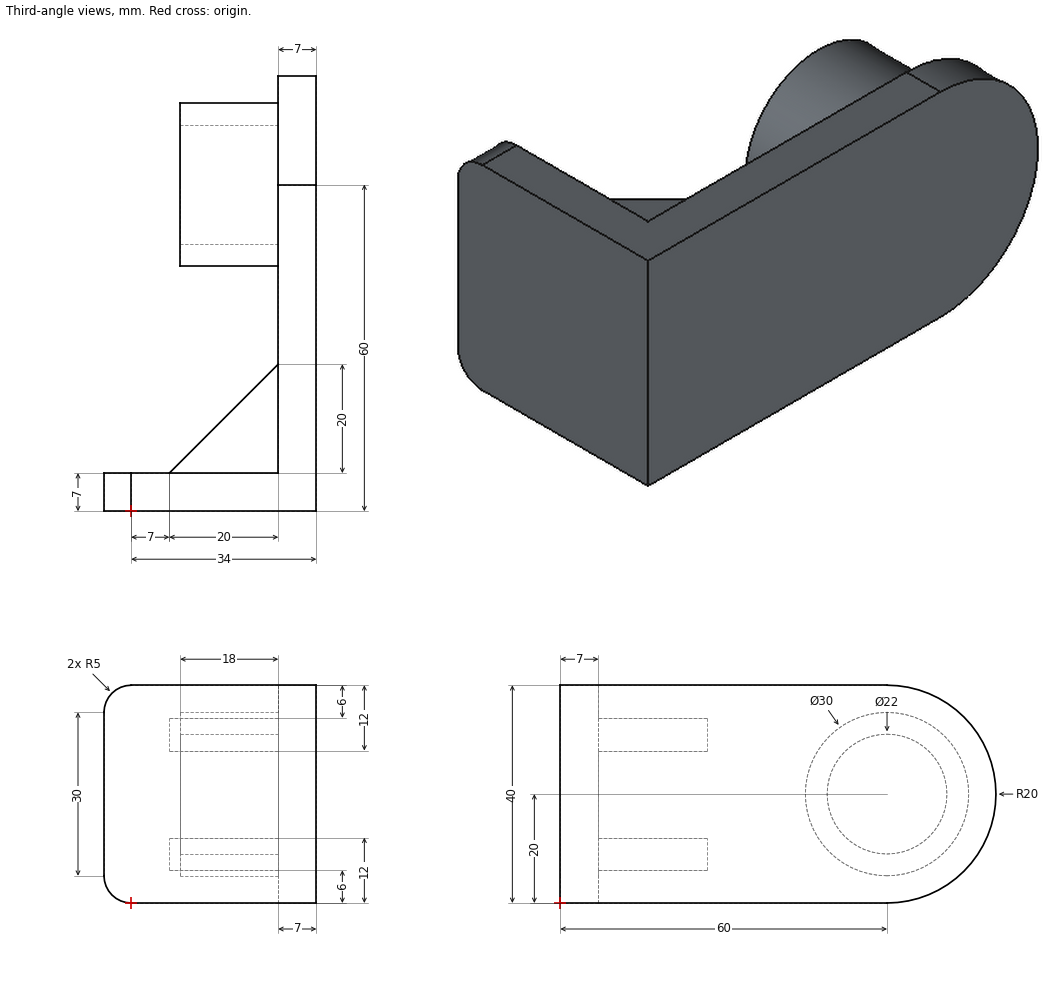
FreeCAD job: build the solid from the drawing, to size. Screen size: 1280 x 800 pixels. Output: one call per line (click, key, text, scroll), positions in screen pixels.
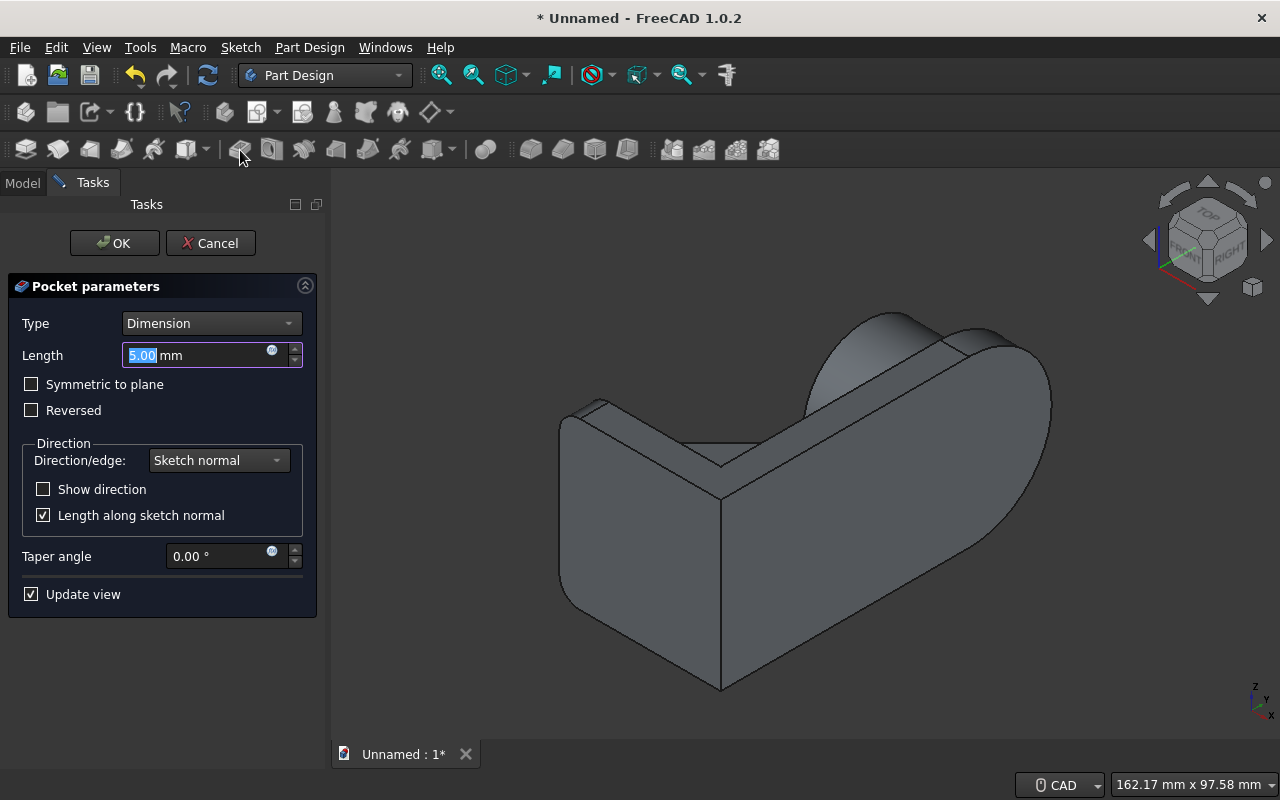
text(6)
key(Tab)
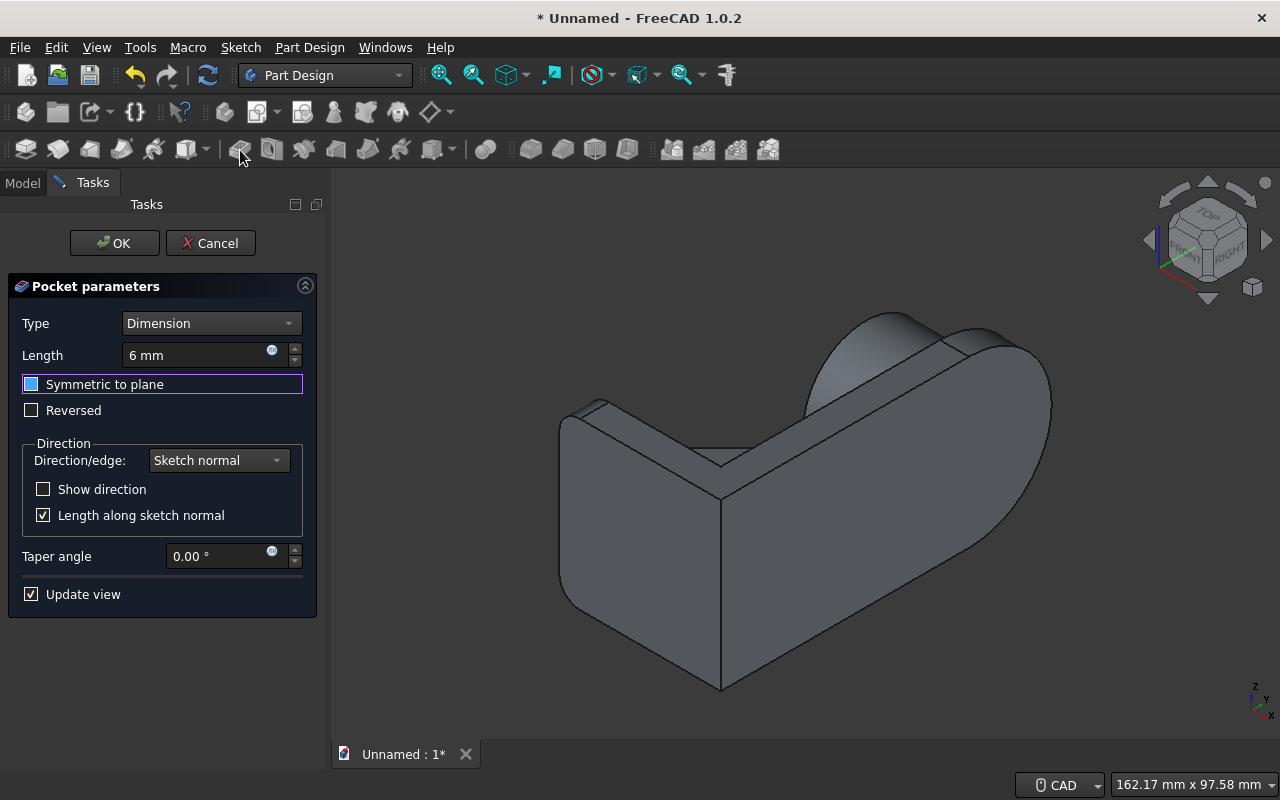
click(115, 243)